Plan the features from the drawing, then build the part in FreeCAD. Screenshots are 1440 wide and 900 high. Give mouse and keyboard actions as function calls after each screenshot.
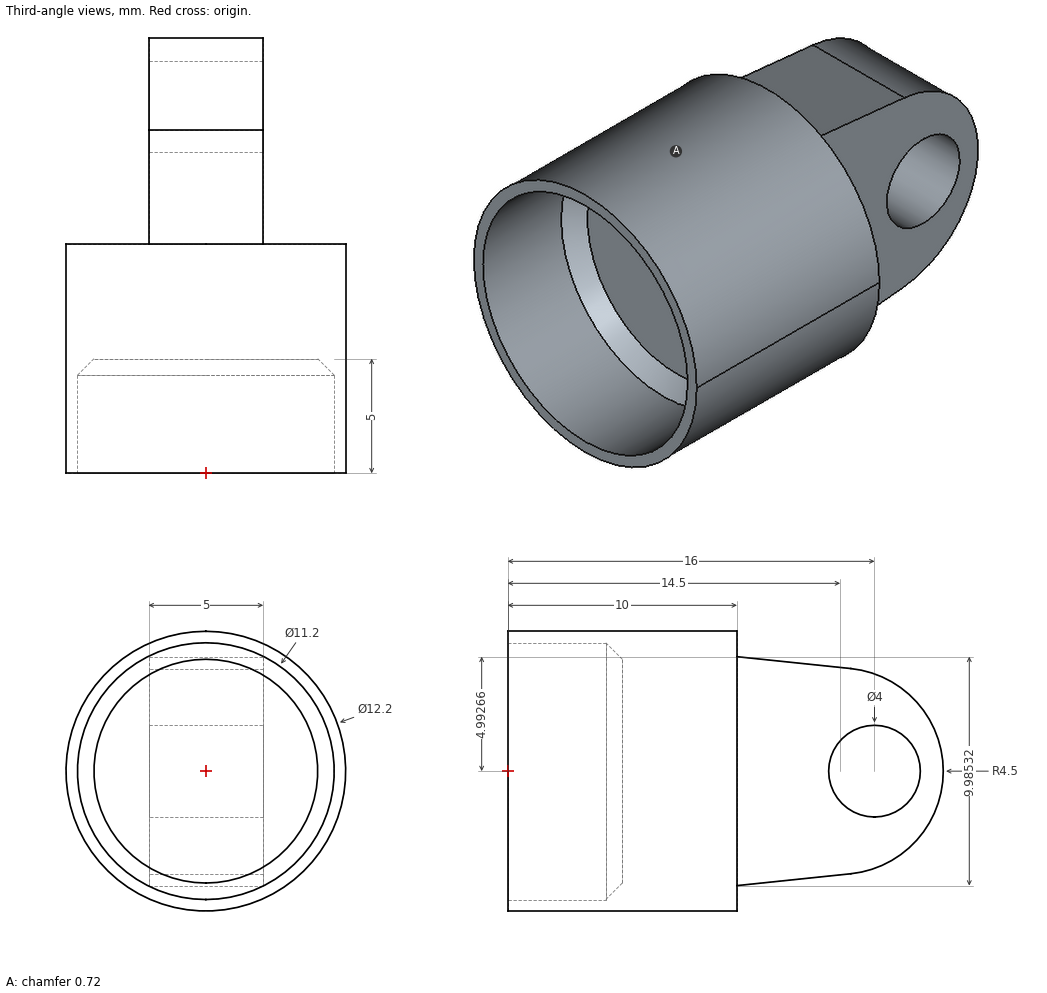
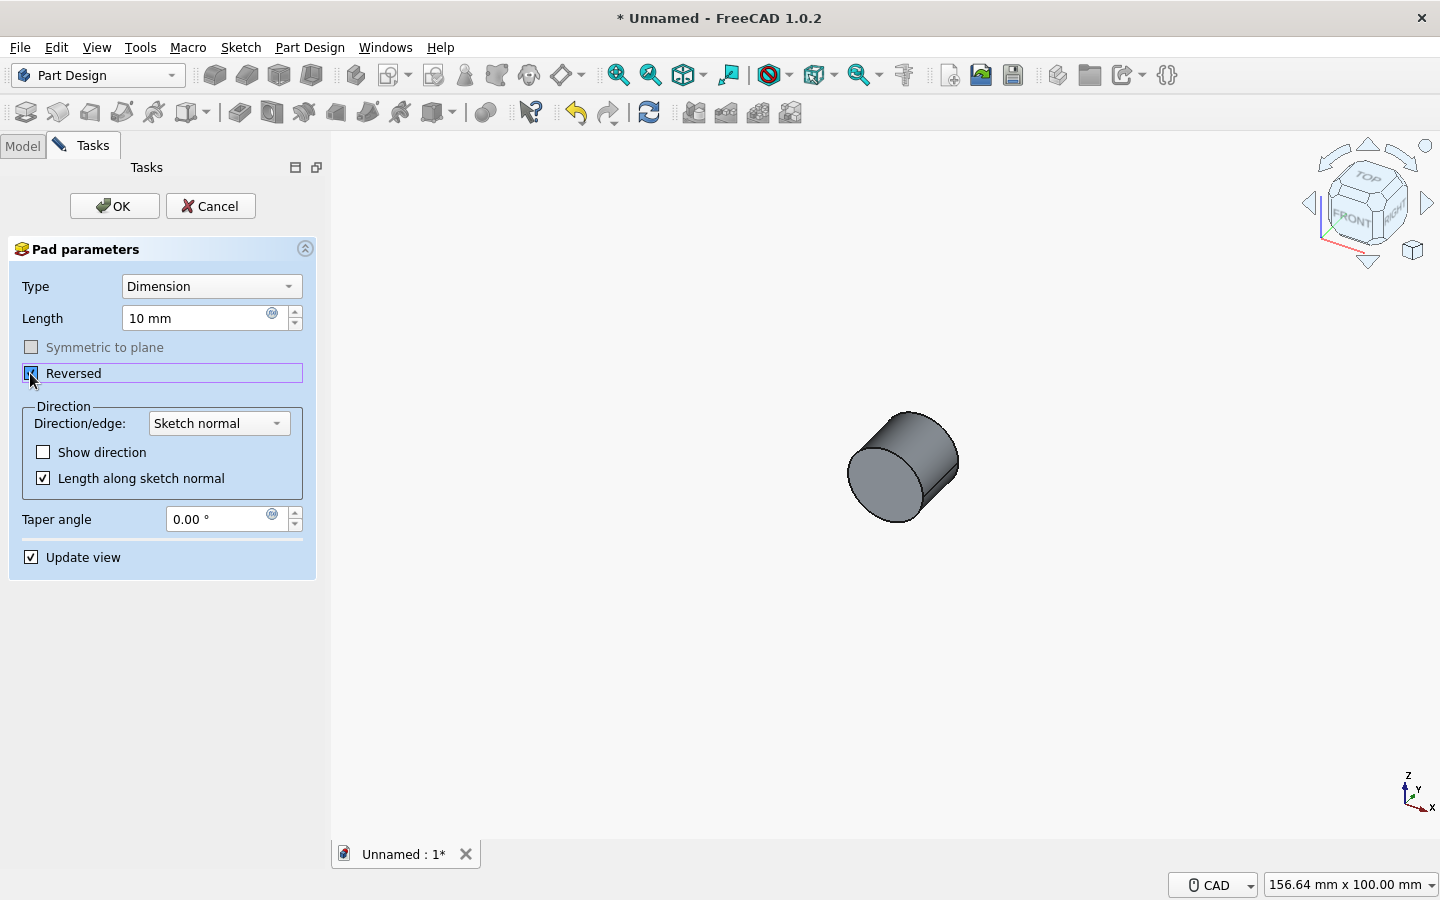
click(115, 206)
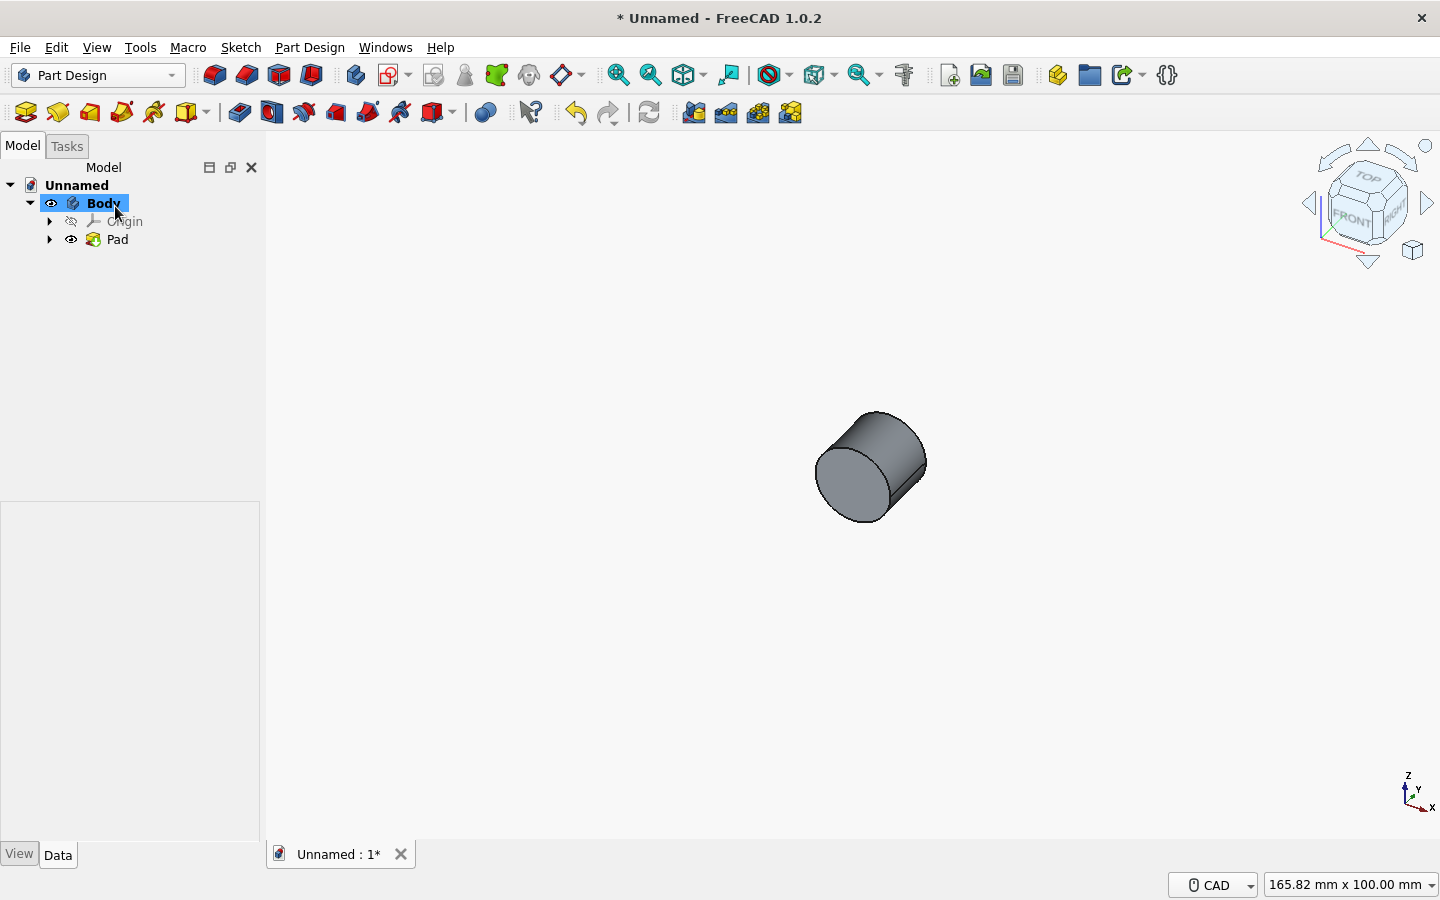
click(620, 76)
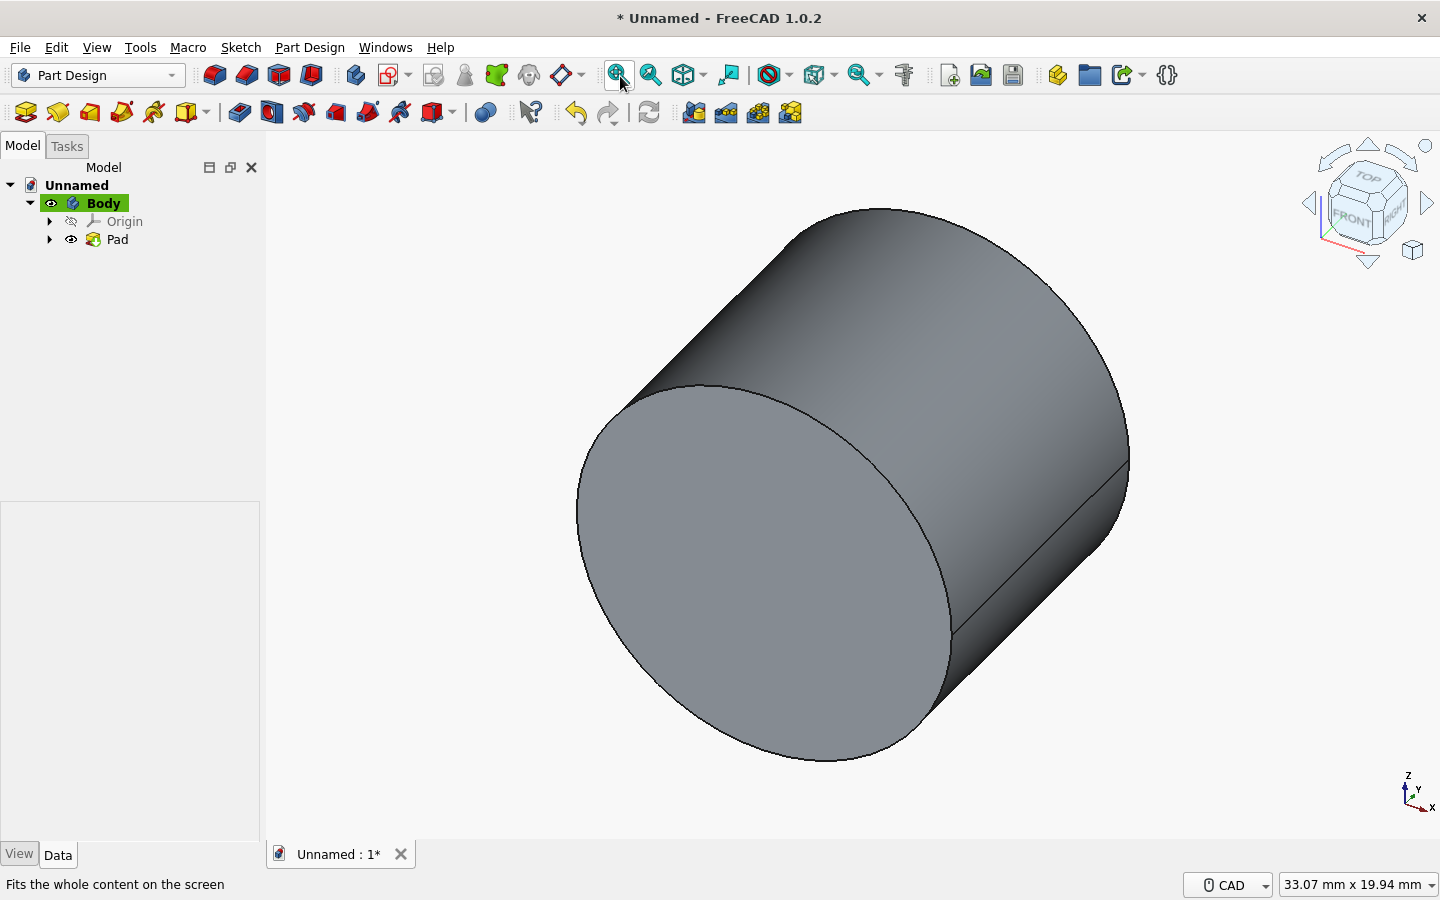
click(388, 76)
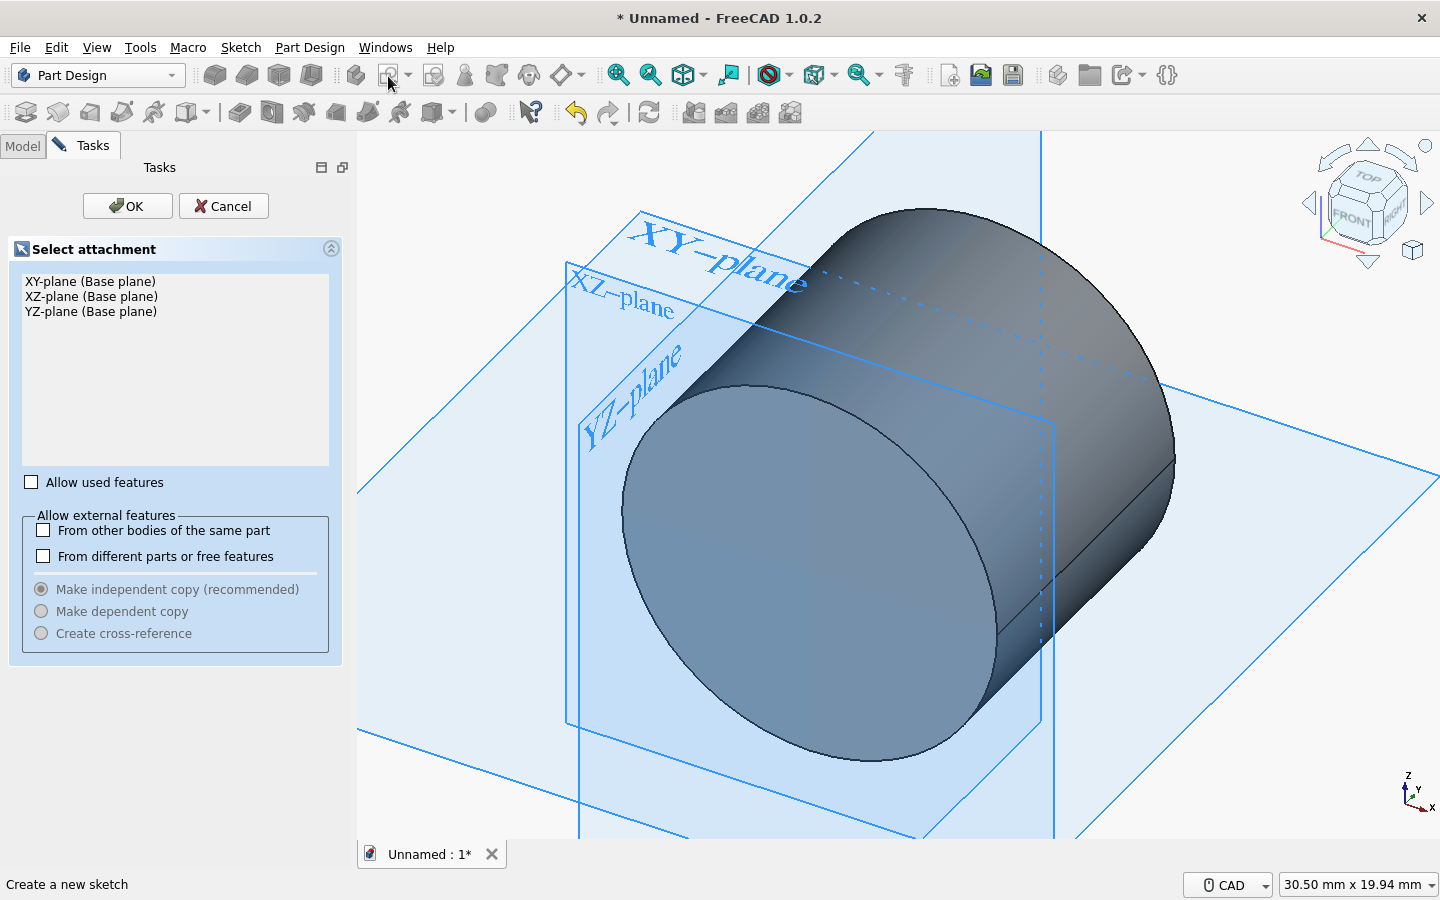
click(82, 312)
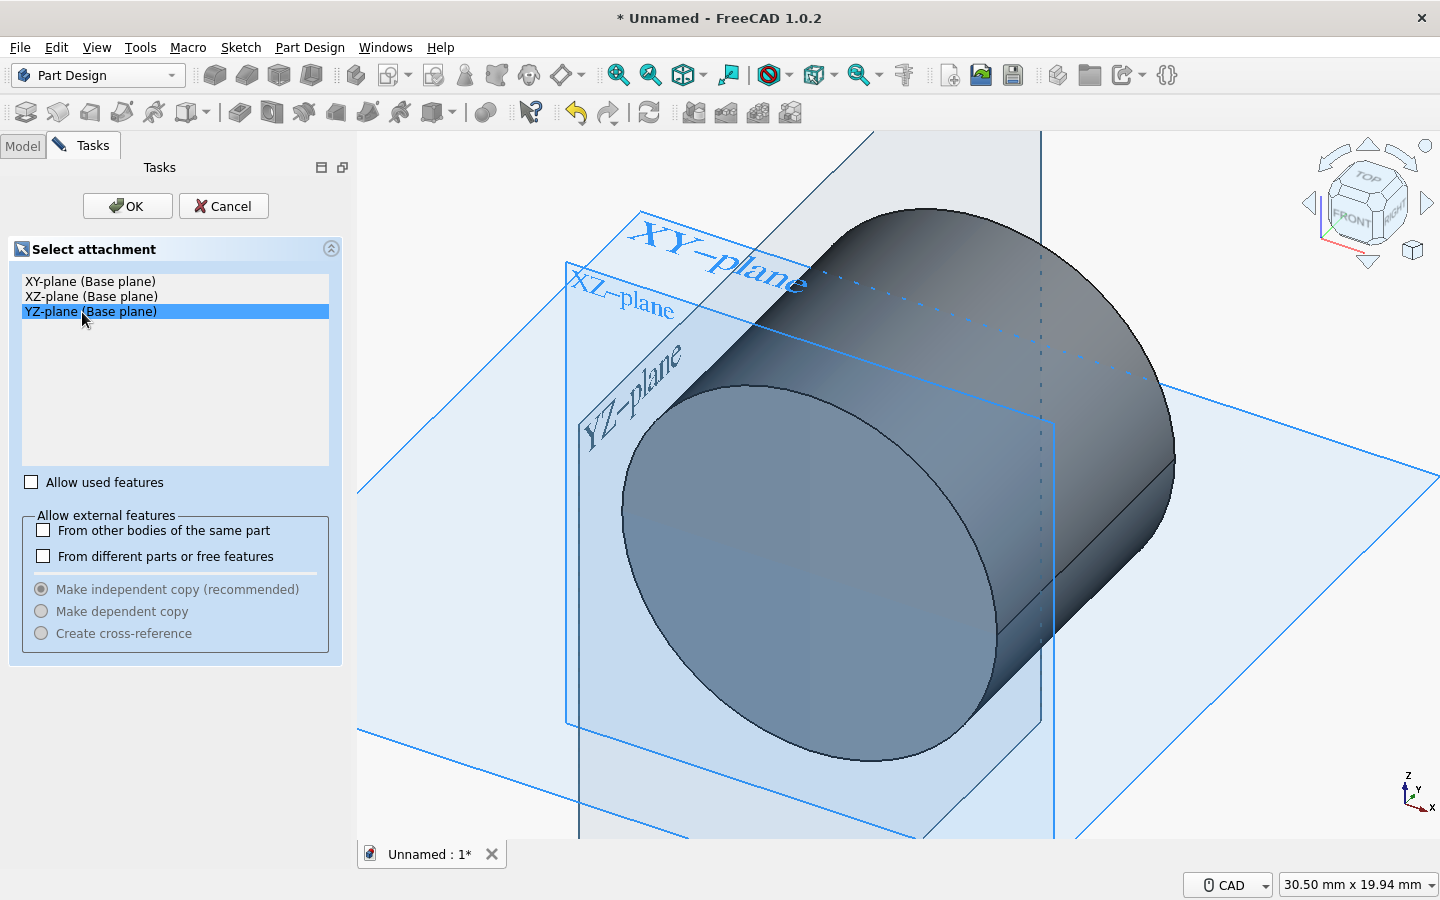
click(128, 206)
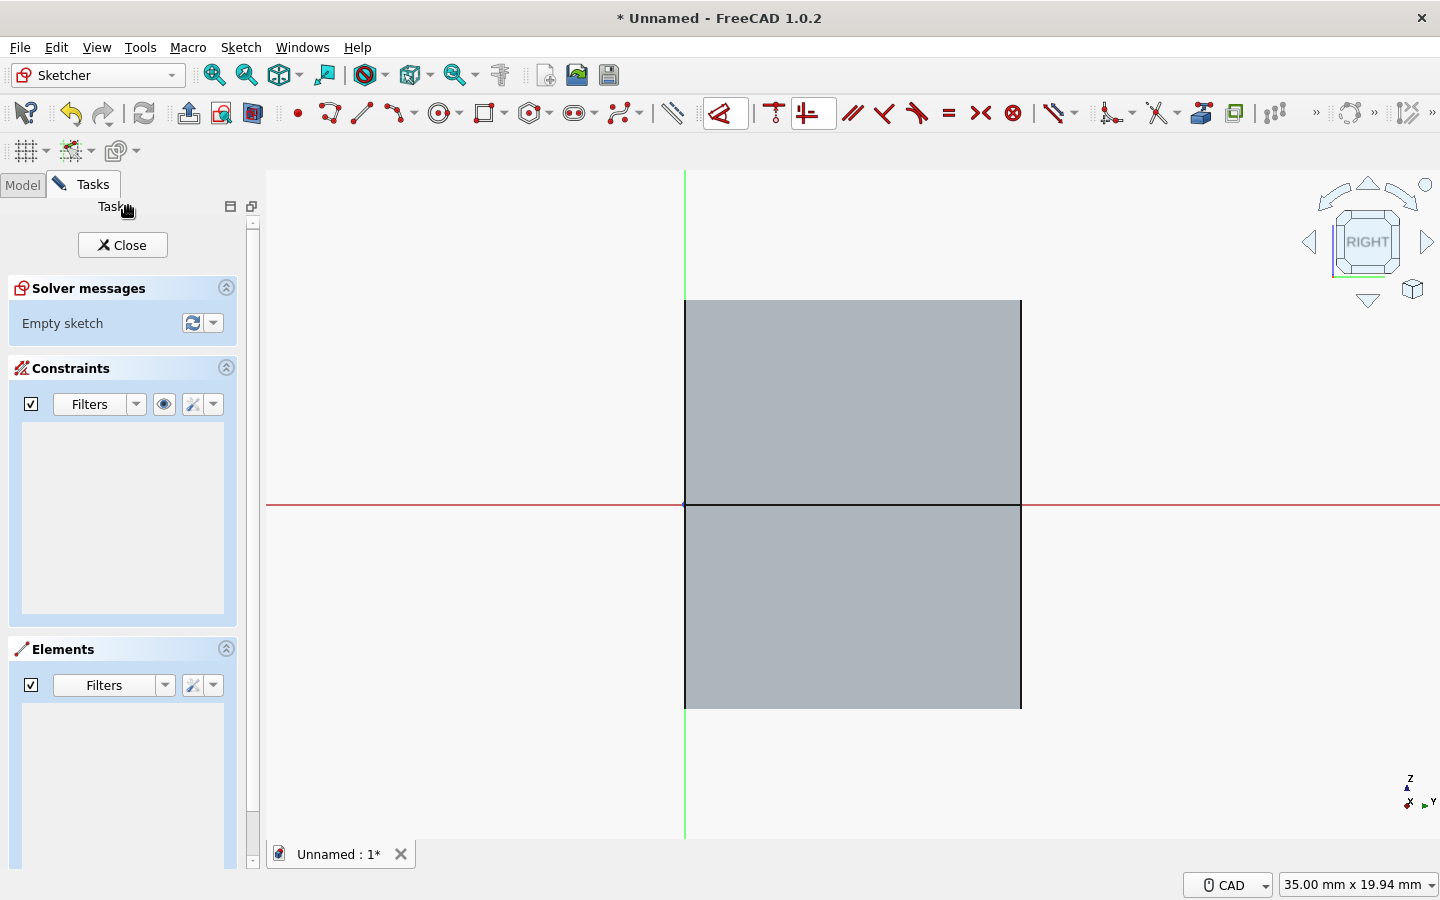
key(q)
key(s)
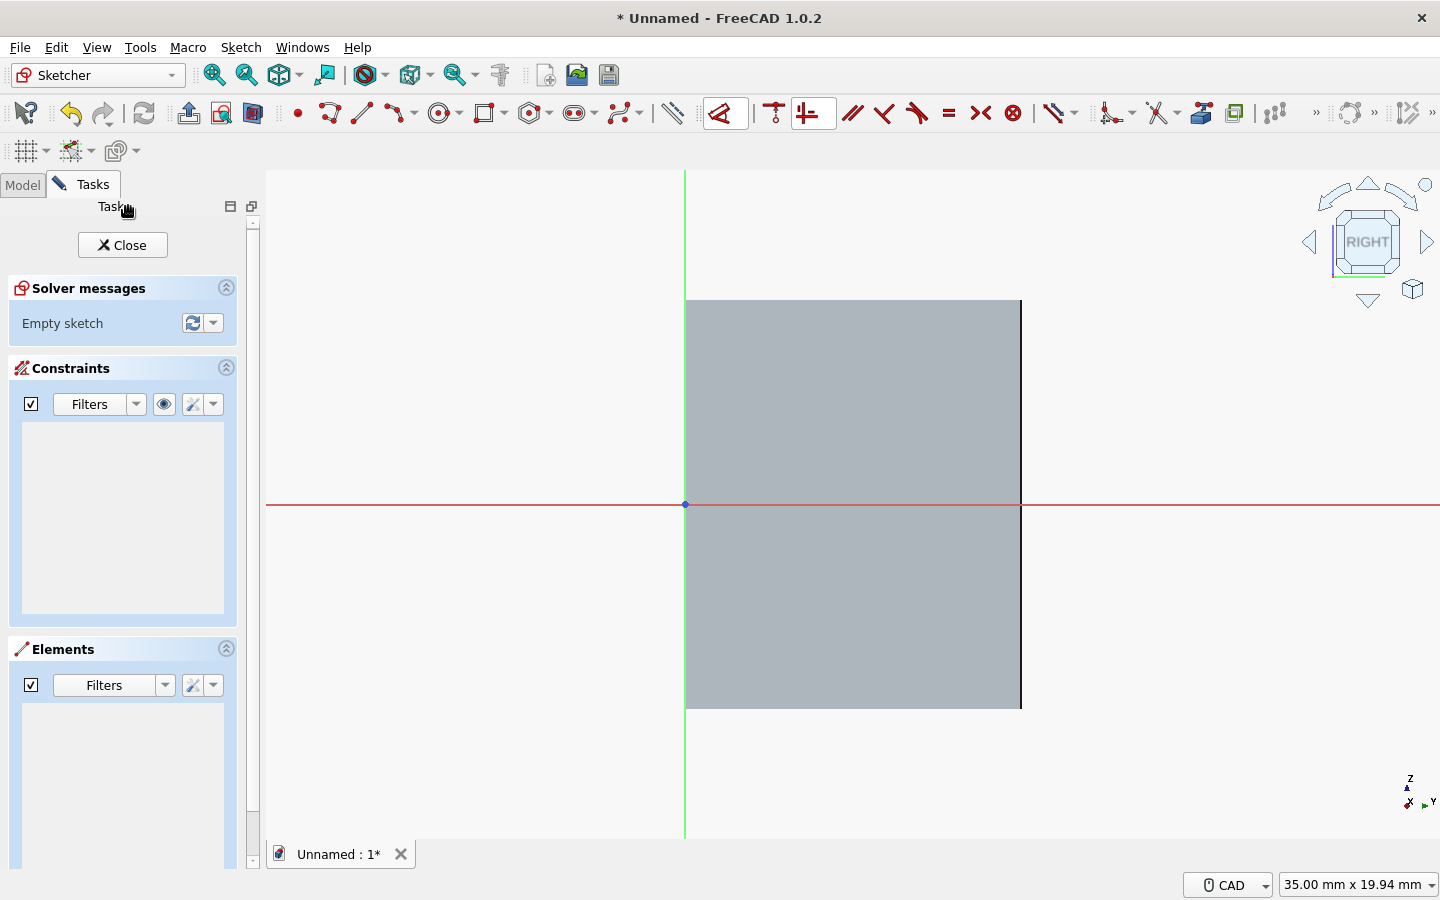
scroll(294, 504, down, 1)